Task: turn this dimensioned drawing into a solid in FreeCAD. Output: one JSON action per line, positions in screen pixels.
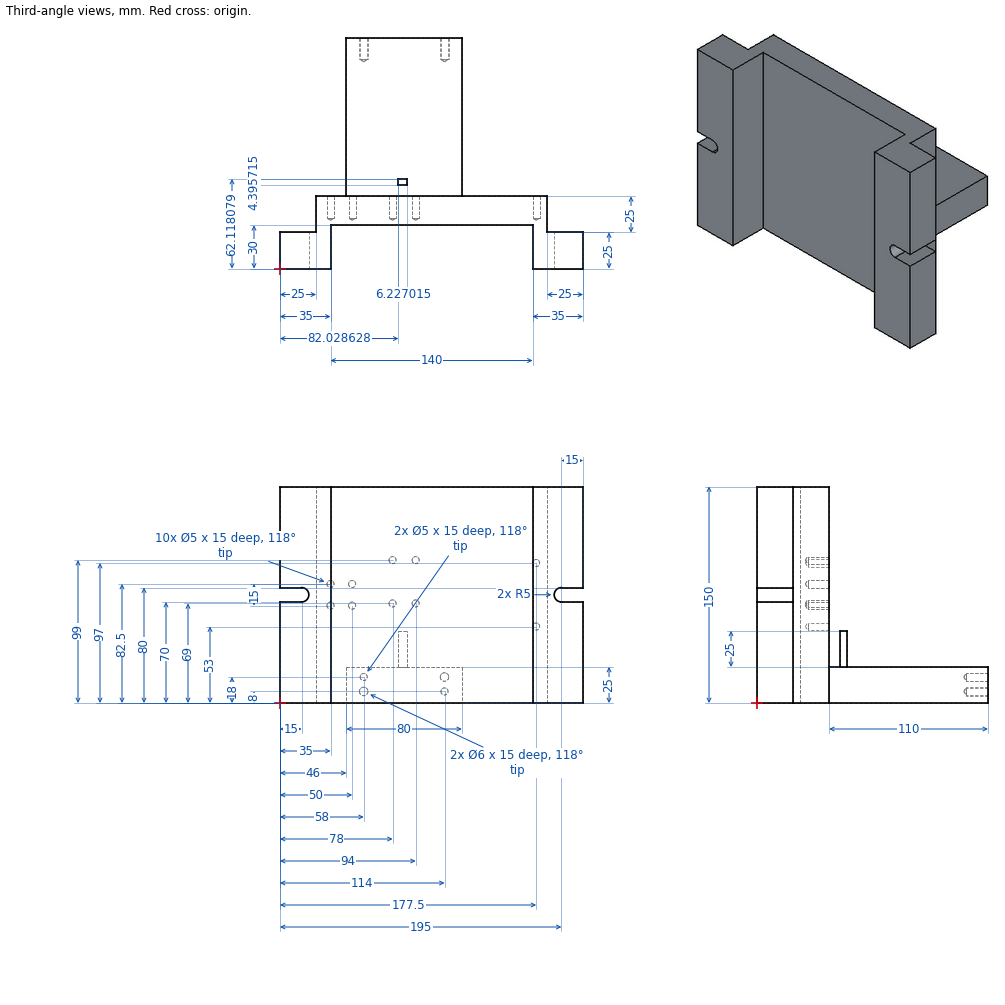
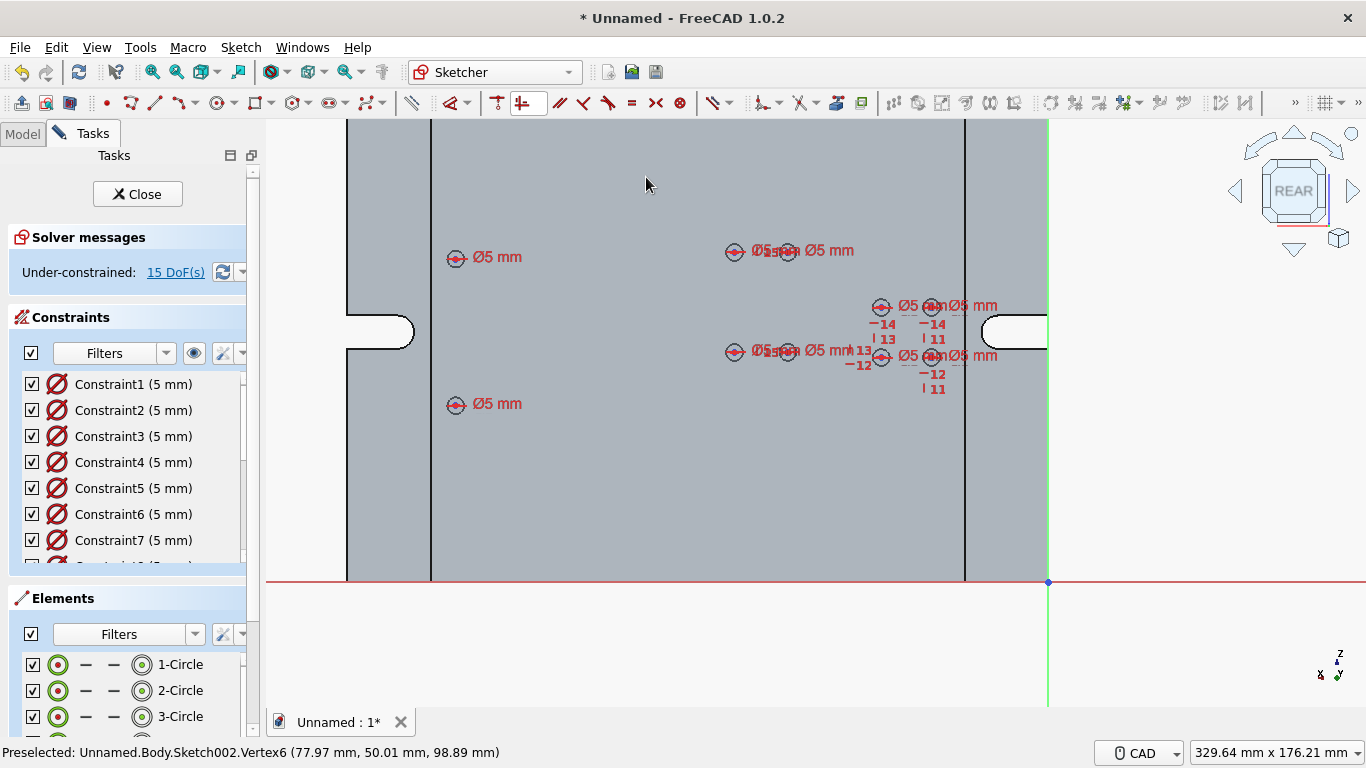
{"action": "left_click", "coordinate": [788, 352]}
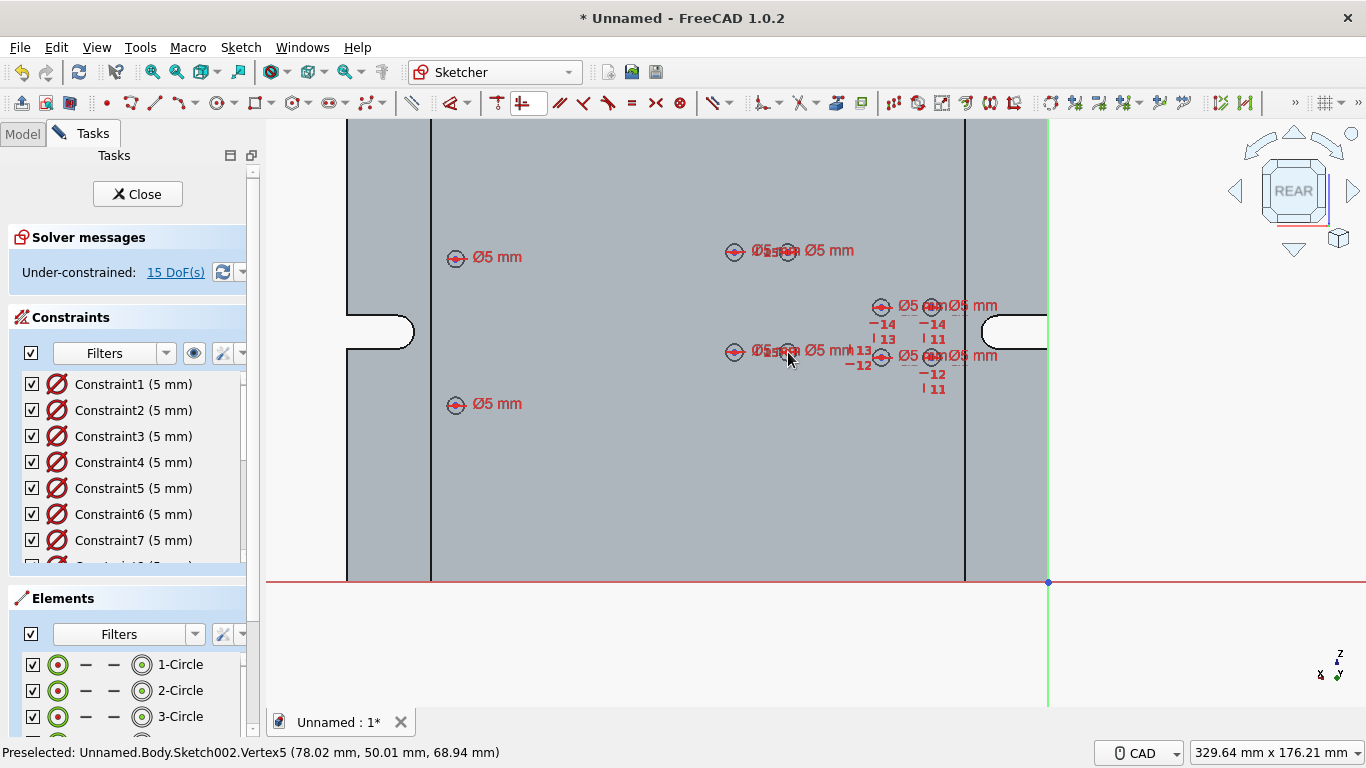
{"action": "left_click", "coordinate": [734, 352]}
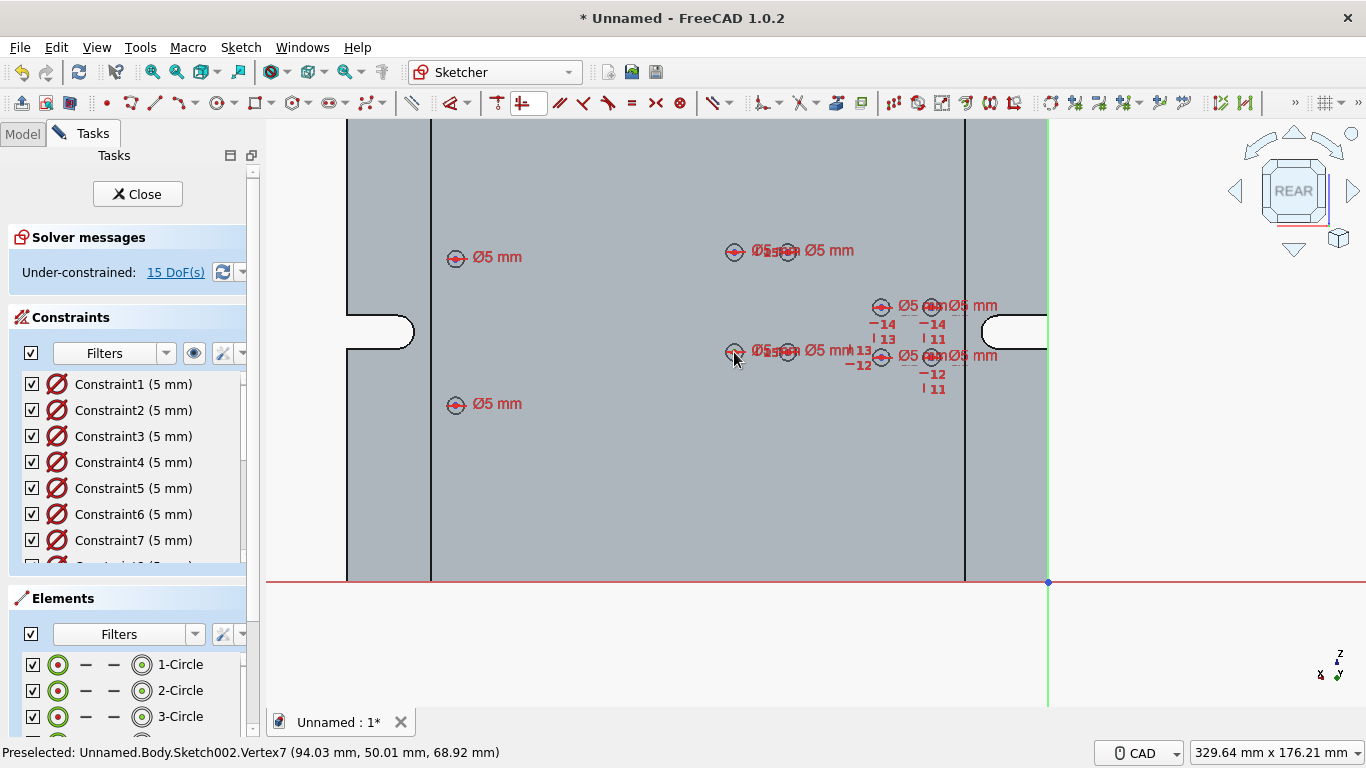
{"action": "key", "text": "h"}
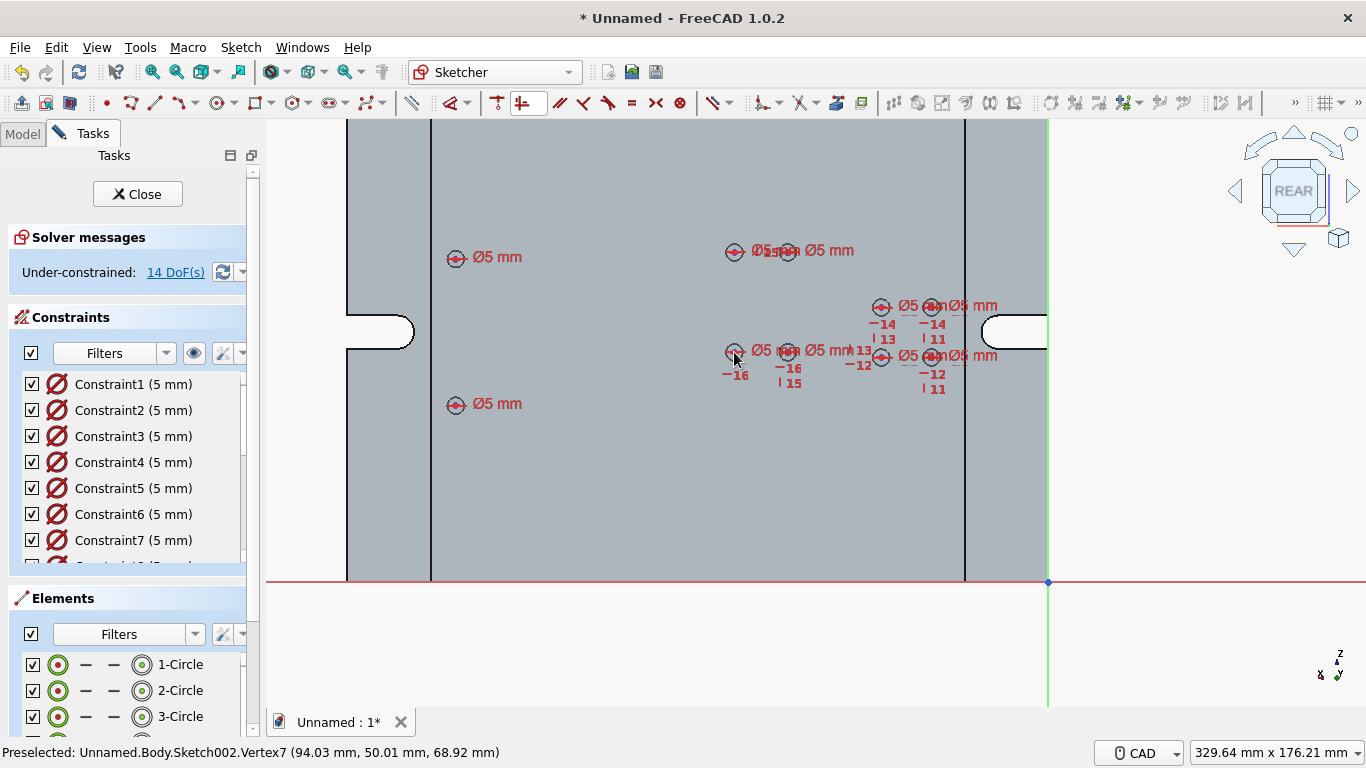
{"action": "left_click", "coordinate": [734, 352]}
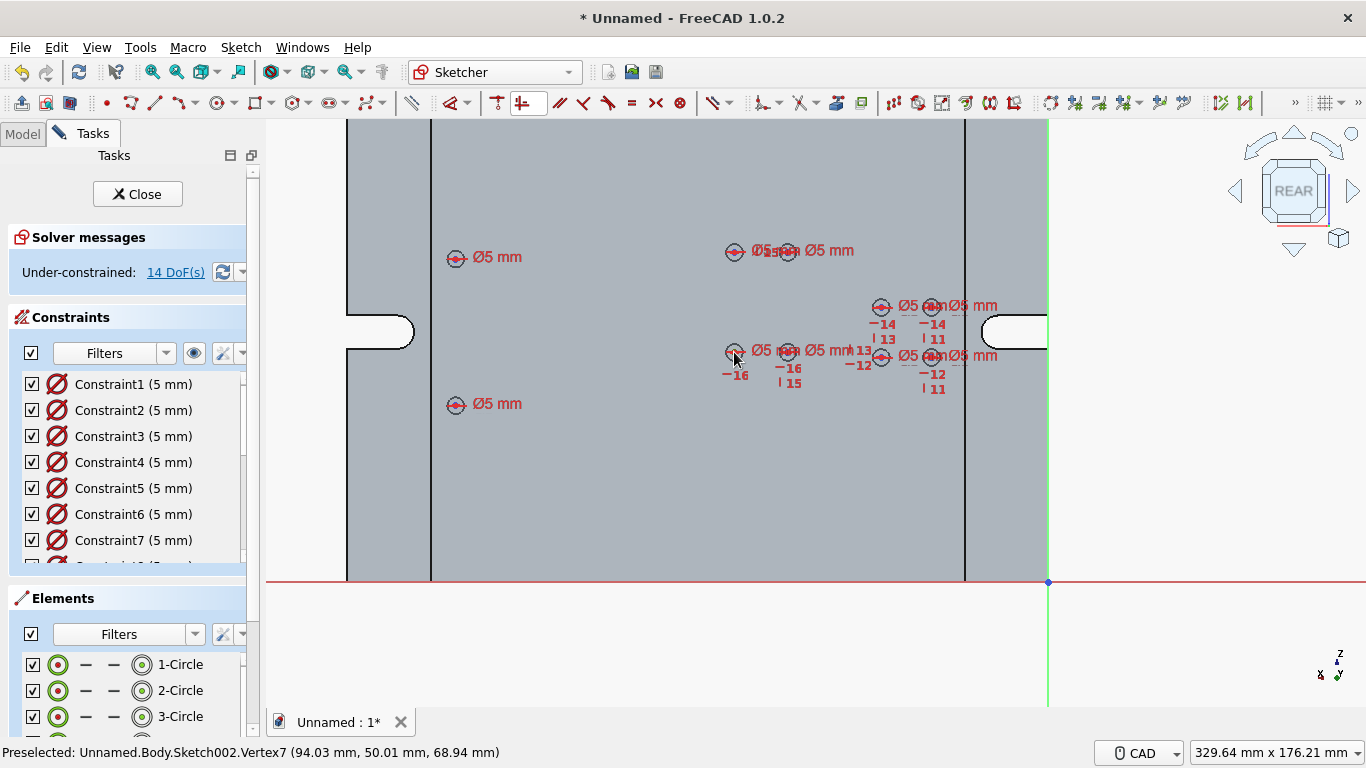
{"action": "left_click", "coordinate": [734, 252]}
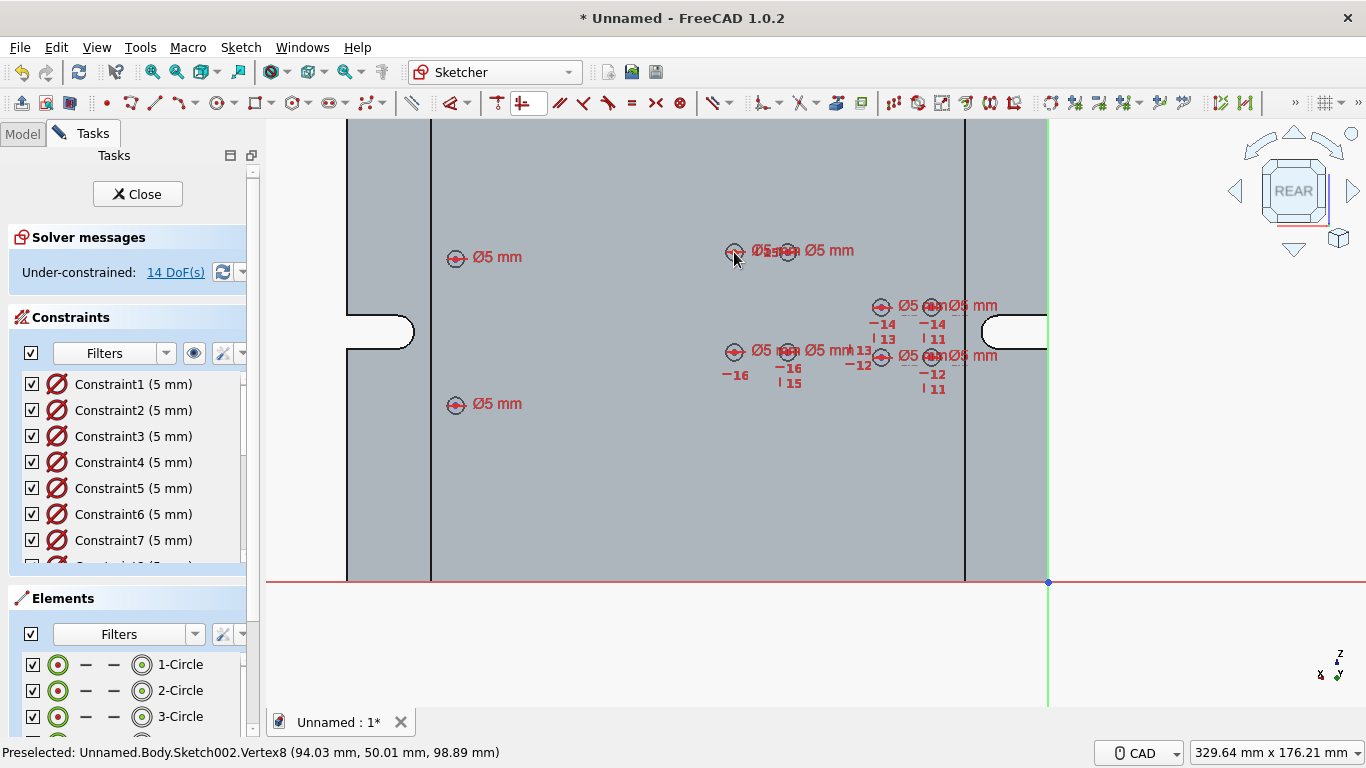
{"action": "key", "text": "v"}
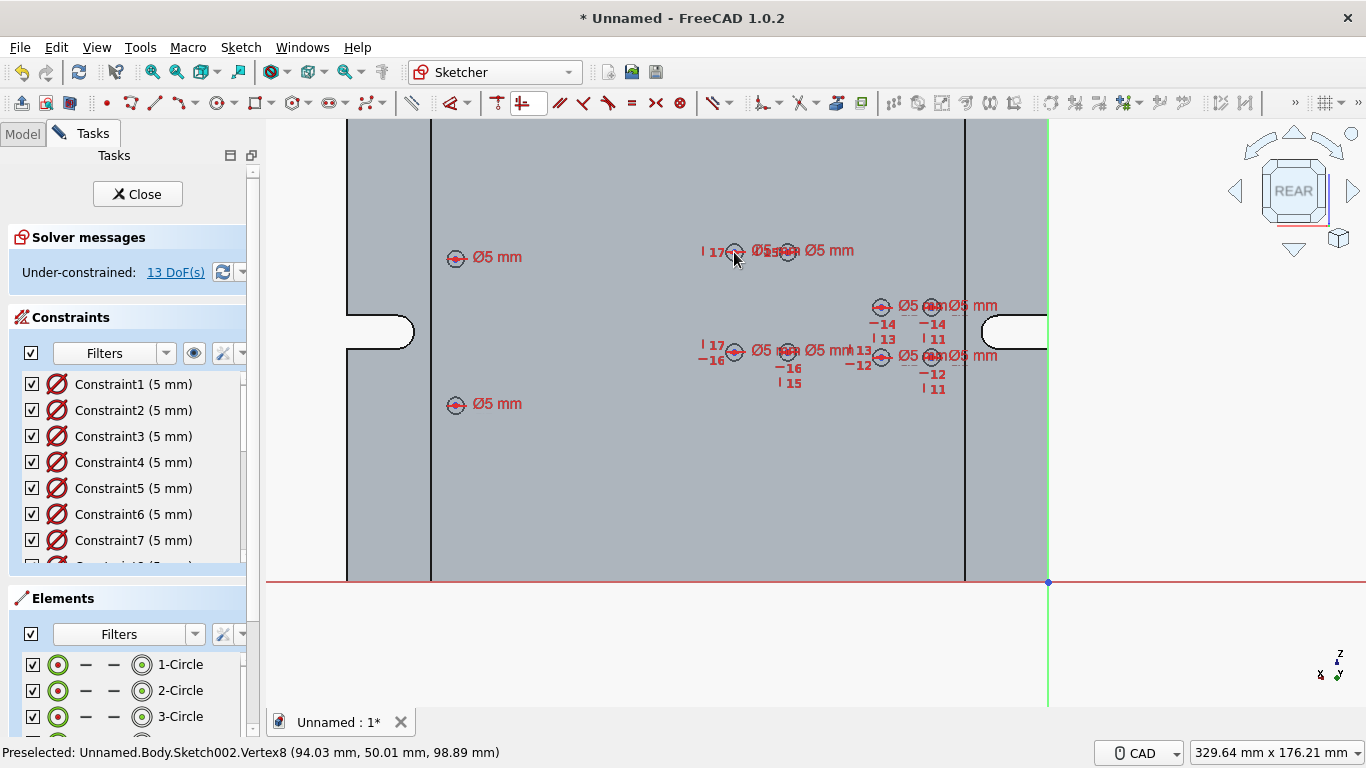
{"action": "left_click", "coordinate": [788, 252]}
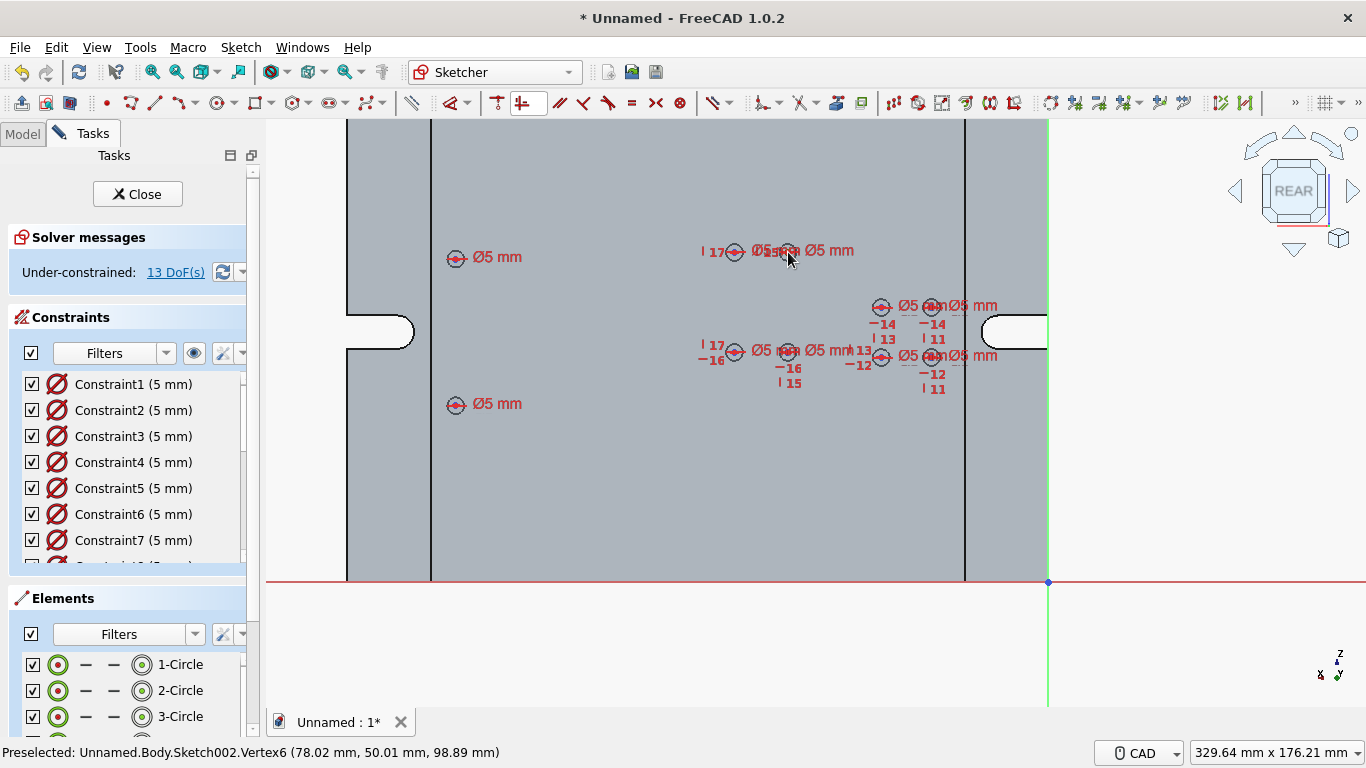
{"action": "left_click", "coordinate": [734, 252]}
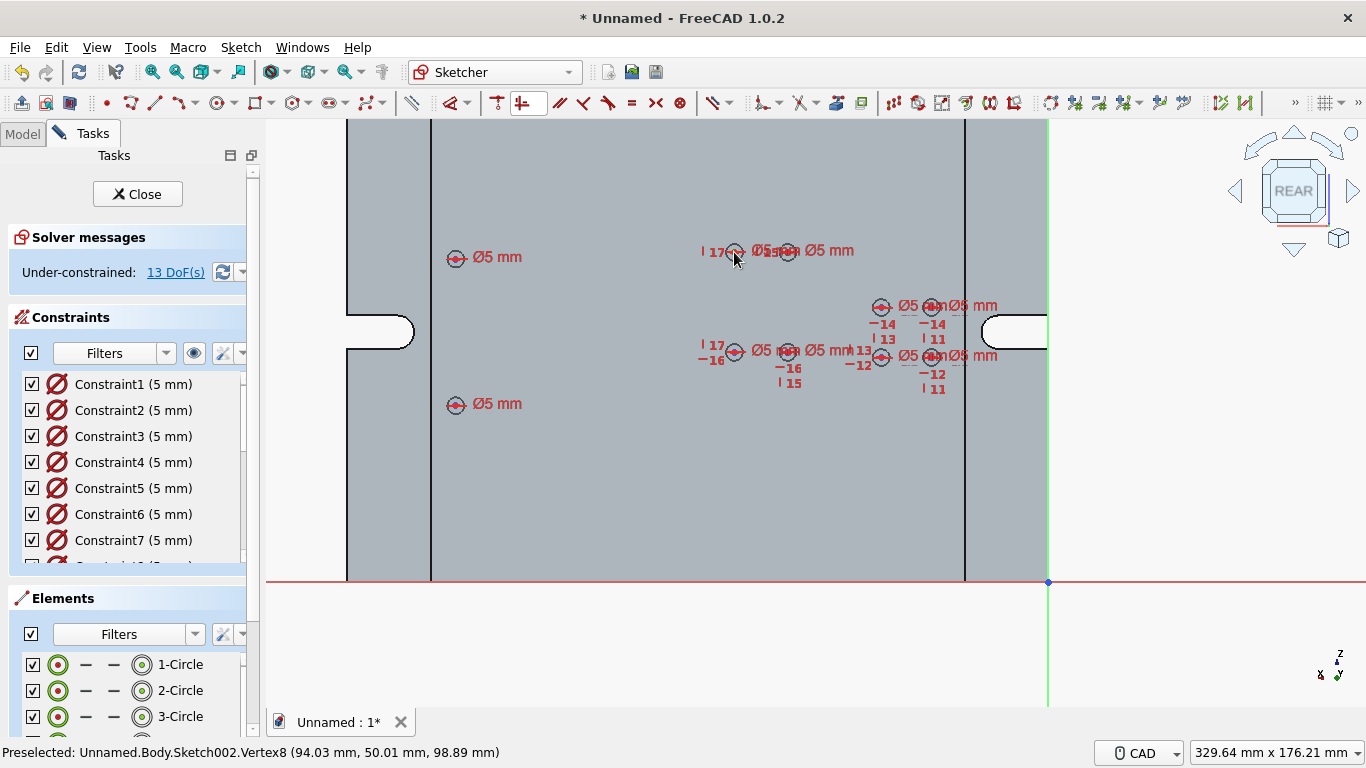
{"action": "key", "text": "h"}